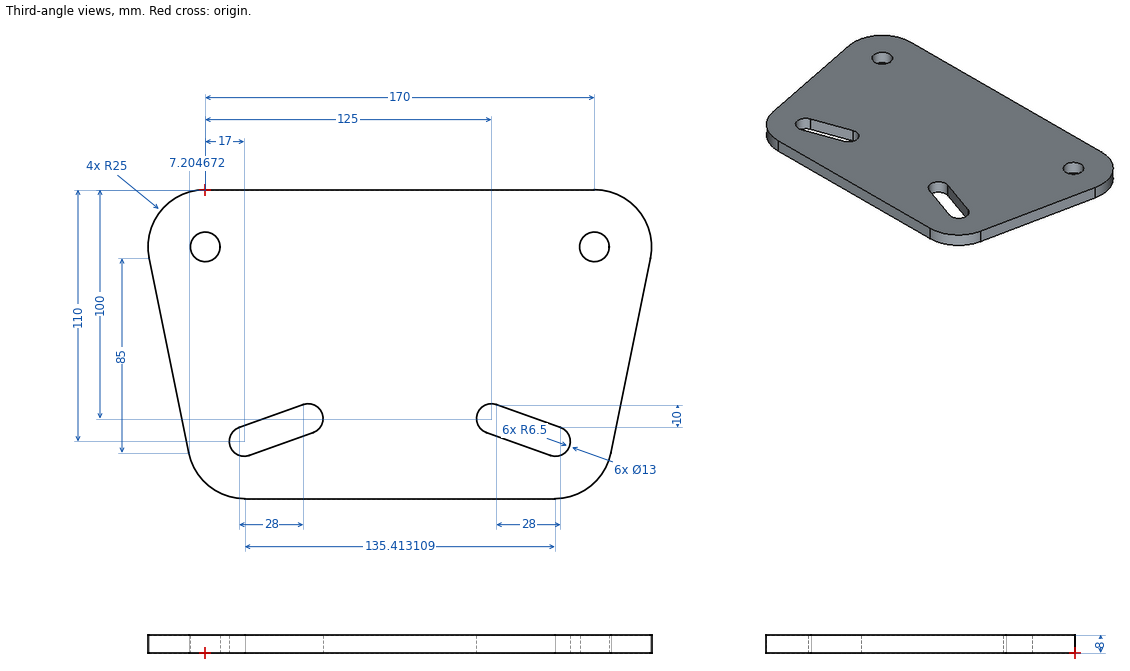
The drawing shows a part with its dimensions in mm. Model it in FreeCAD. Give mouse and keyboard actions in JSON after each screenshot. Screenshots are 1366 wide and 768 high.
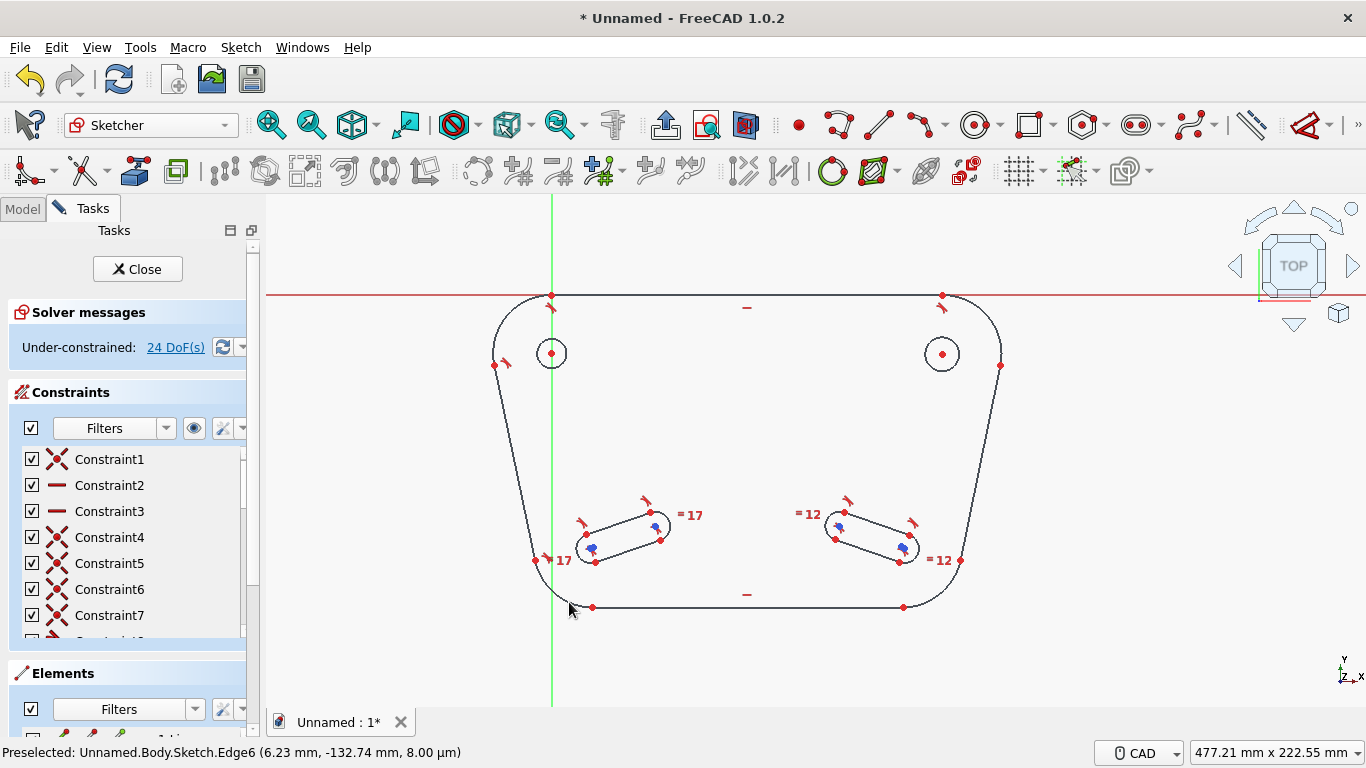
{"action": "left_click", "coordinate": [686, 608]}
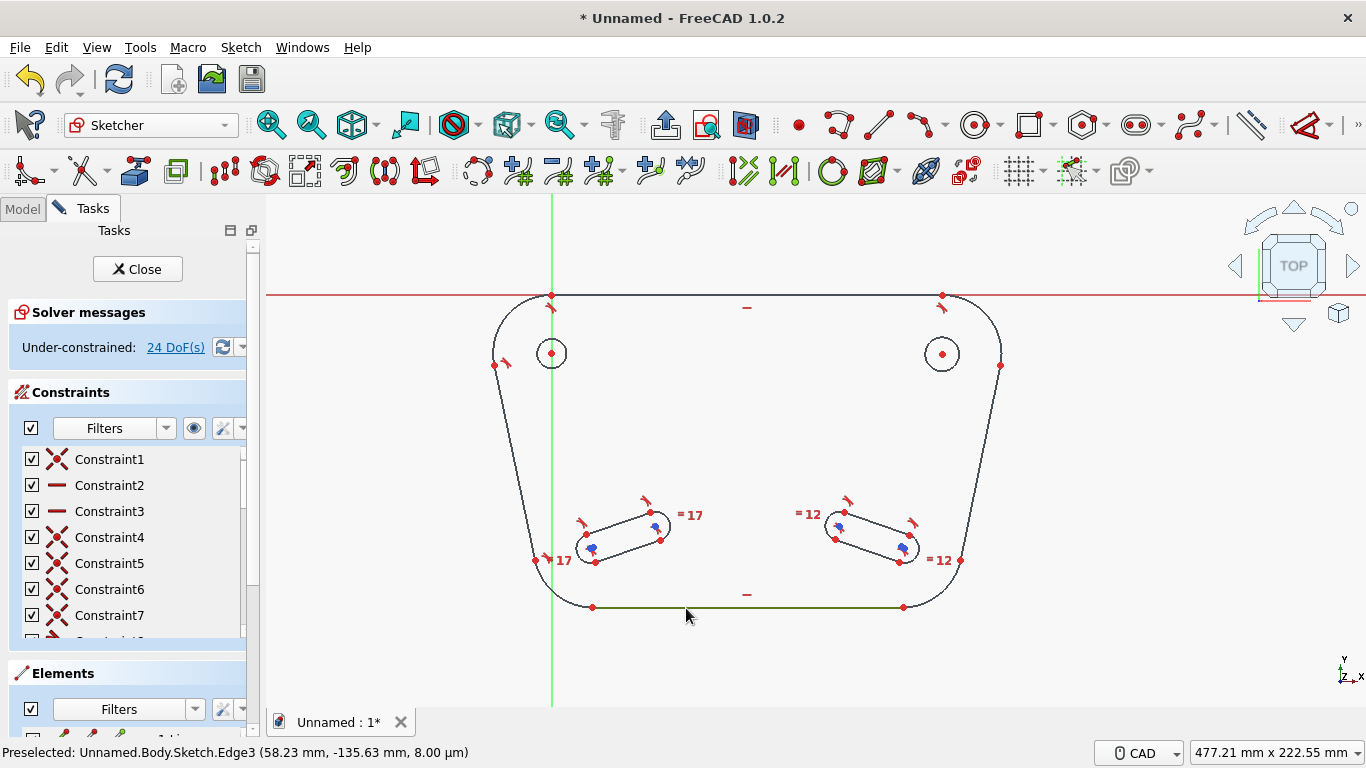
{"action": "left_click", "coordinate": [569, 602]}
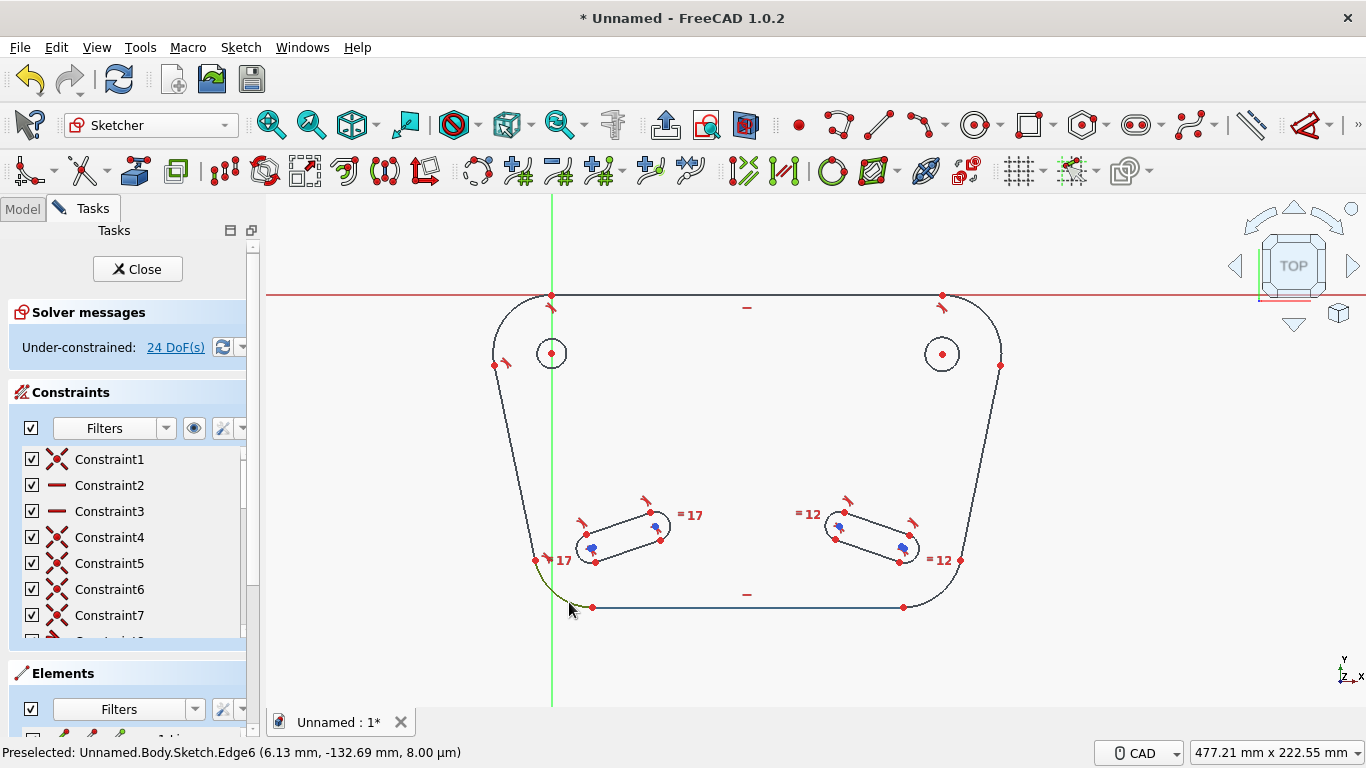
{"action": "key", "text": "t"}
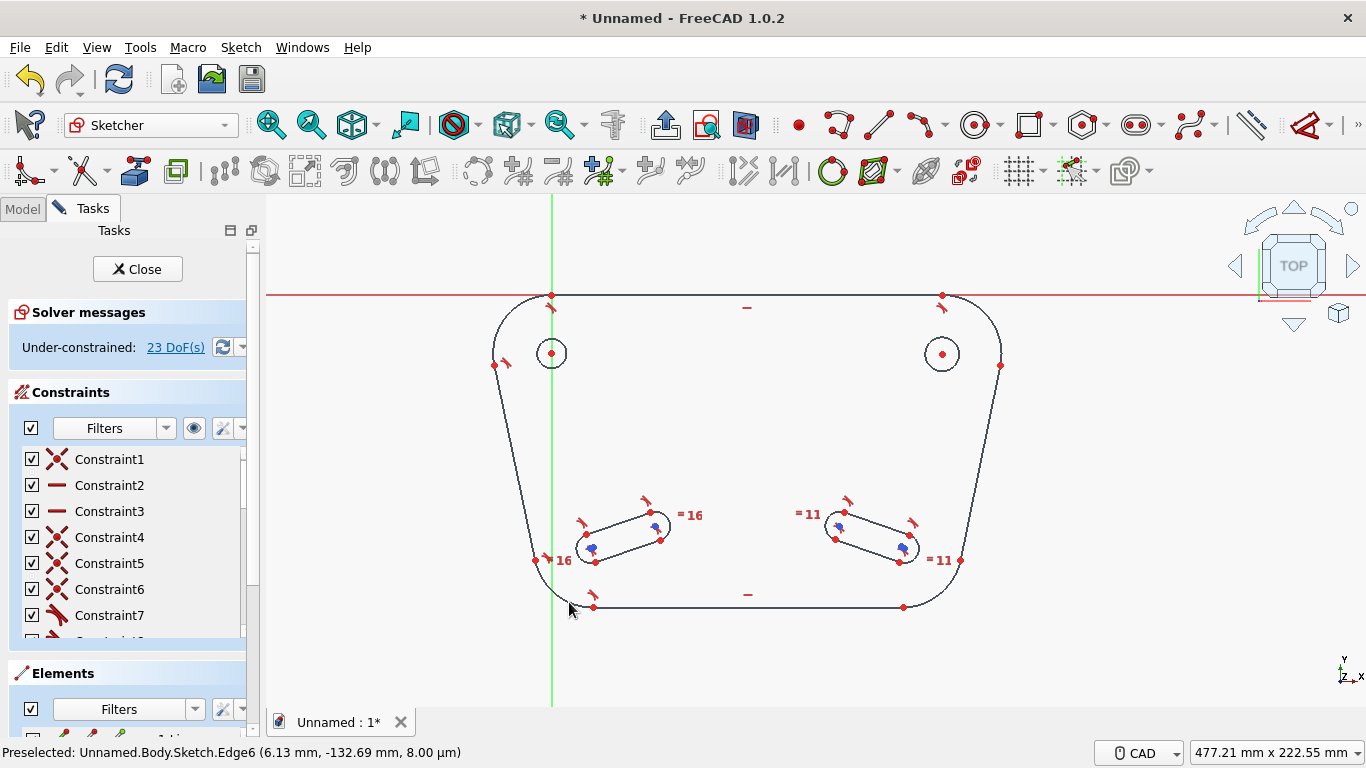
{"action": "left_click", "coordinate": [687, 608]}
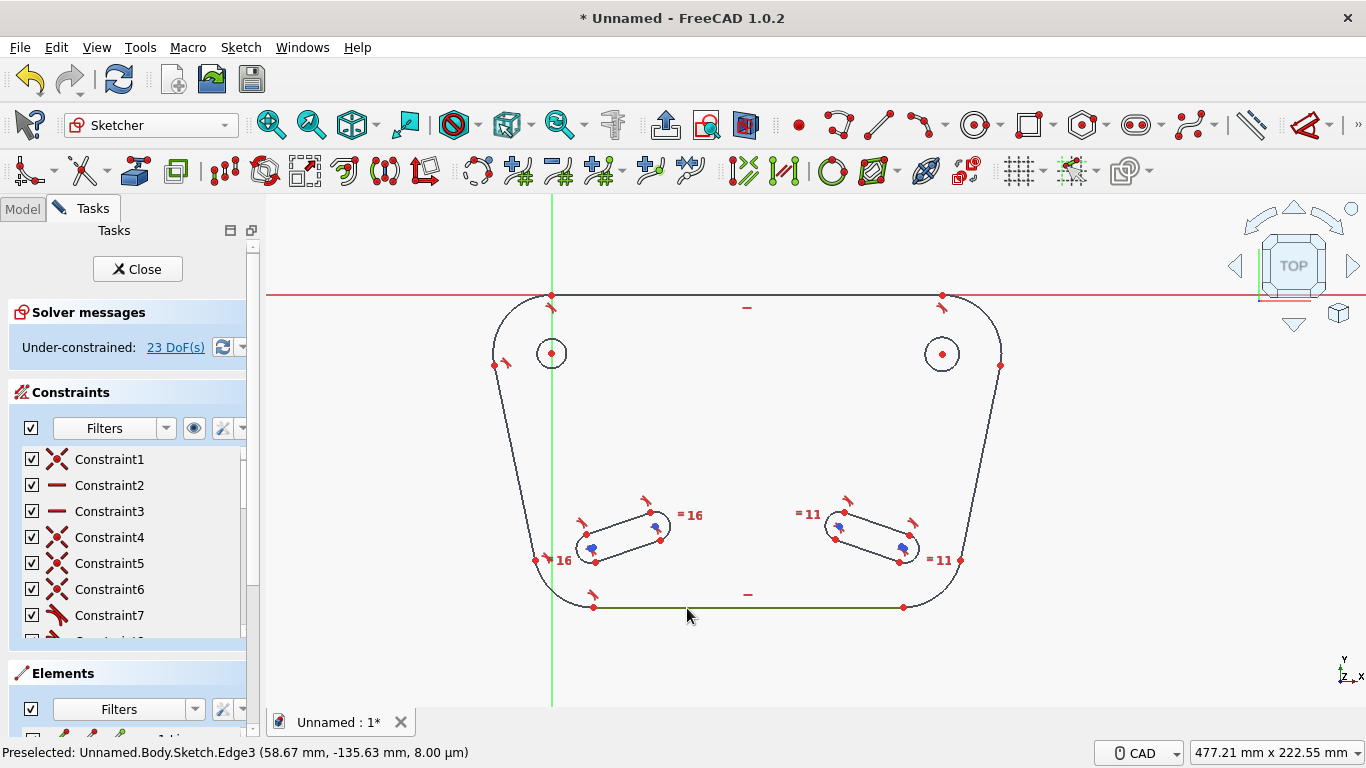
{"action": "left_click", "coordinate": [927, 602]}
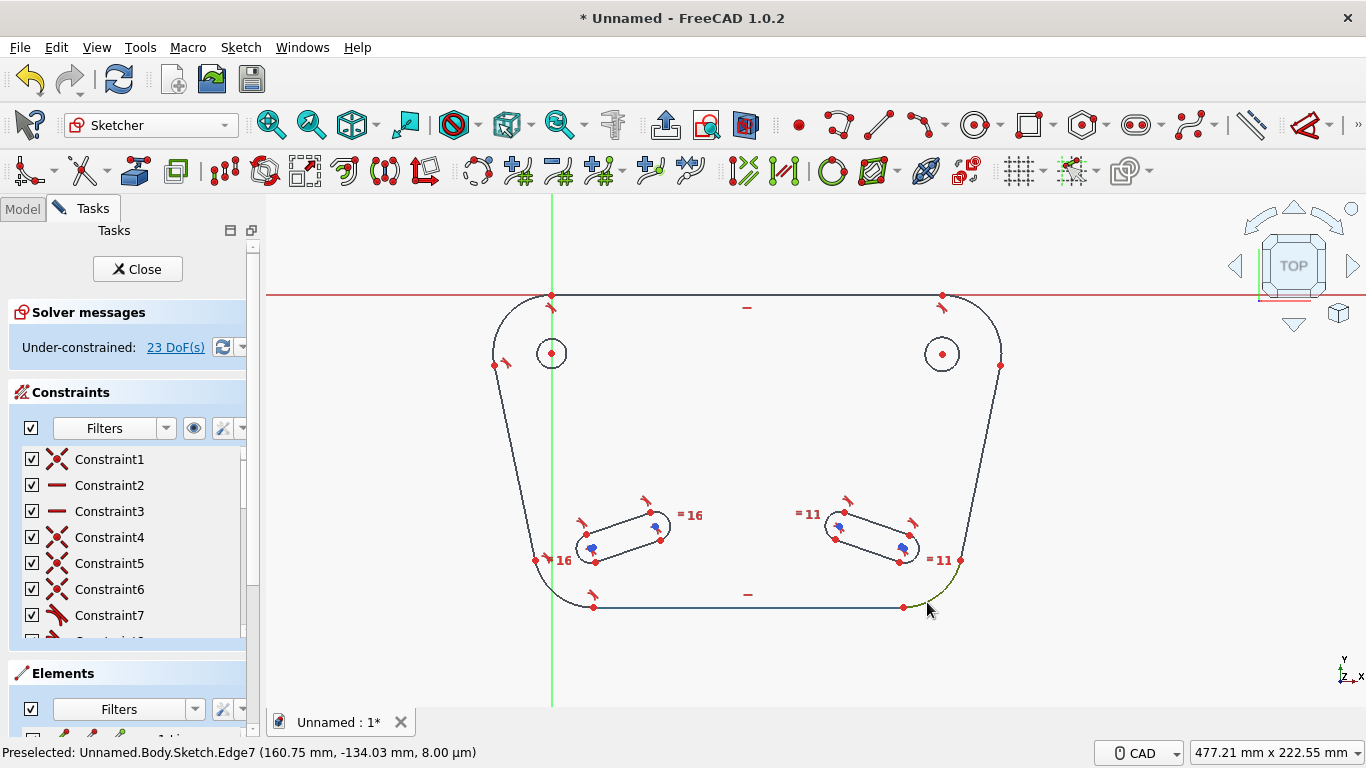
{"action": "key", "text": "t"}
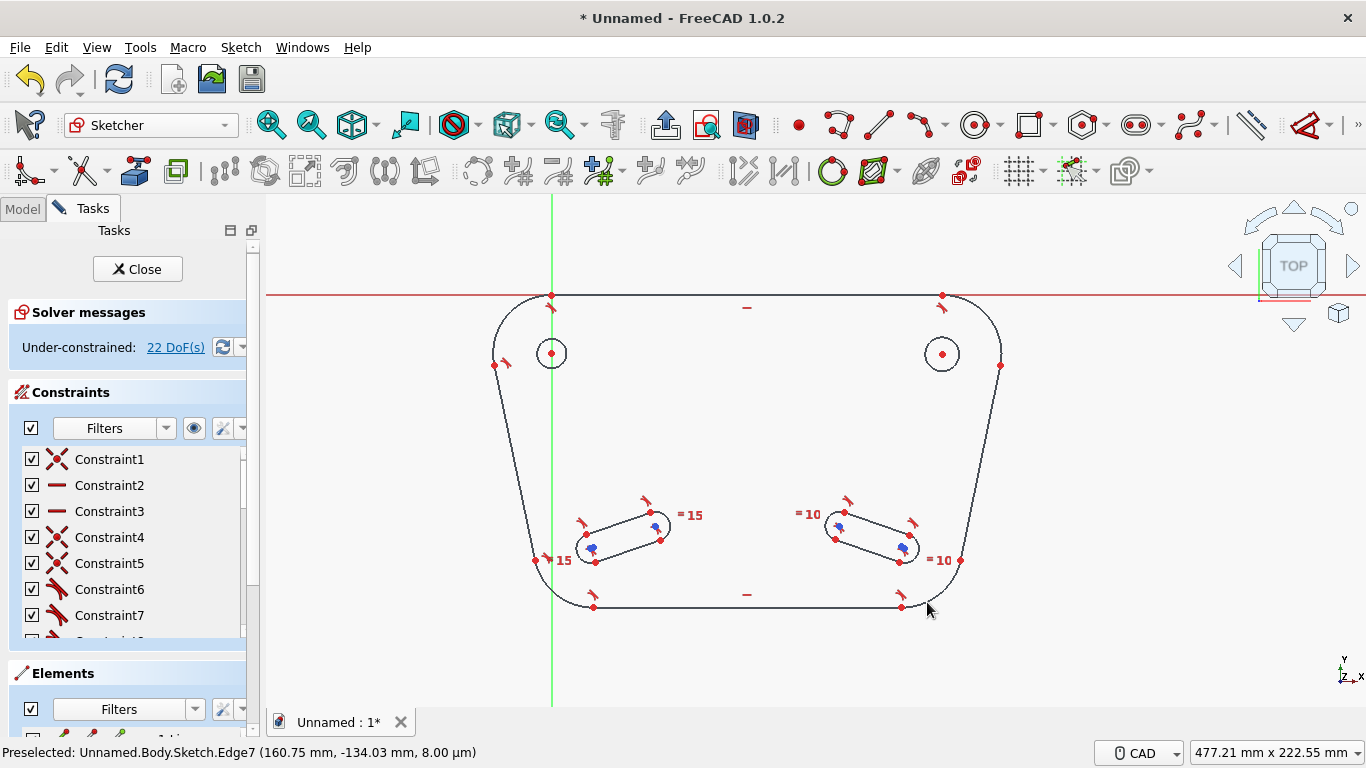
{"action": "left_click", "coordinate": [973, 502]}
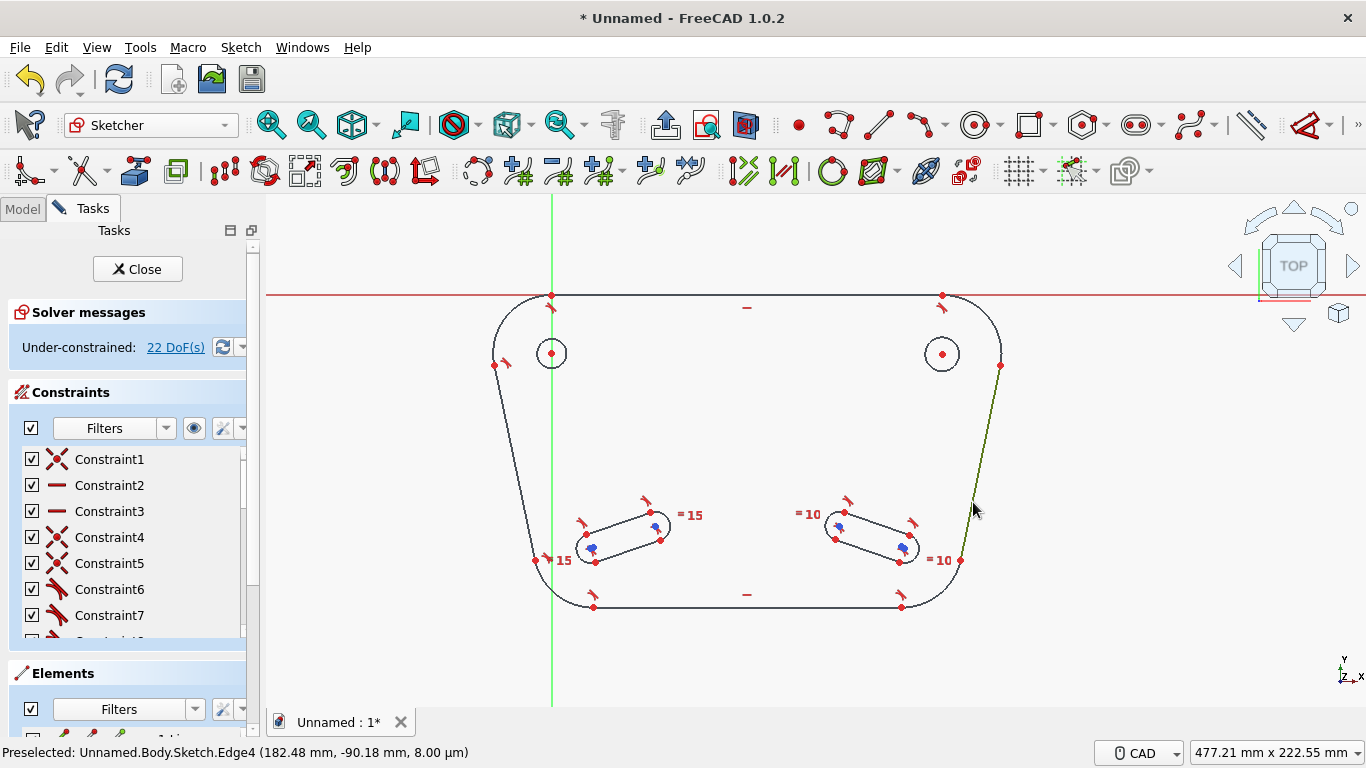
{"action": "left_click", "coordinate": [925, 603]}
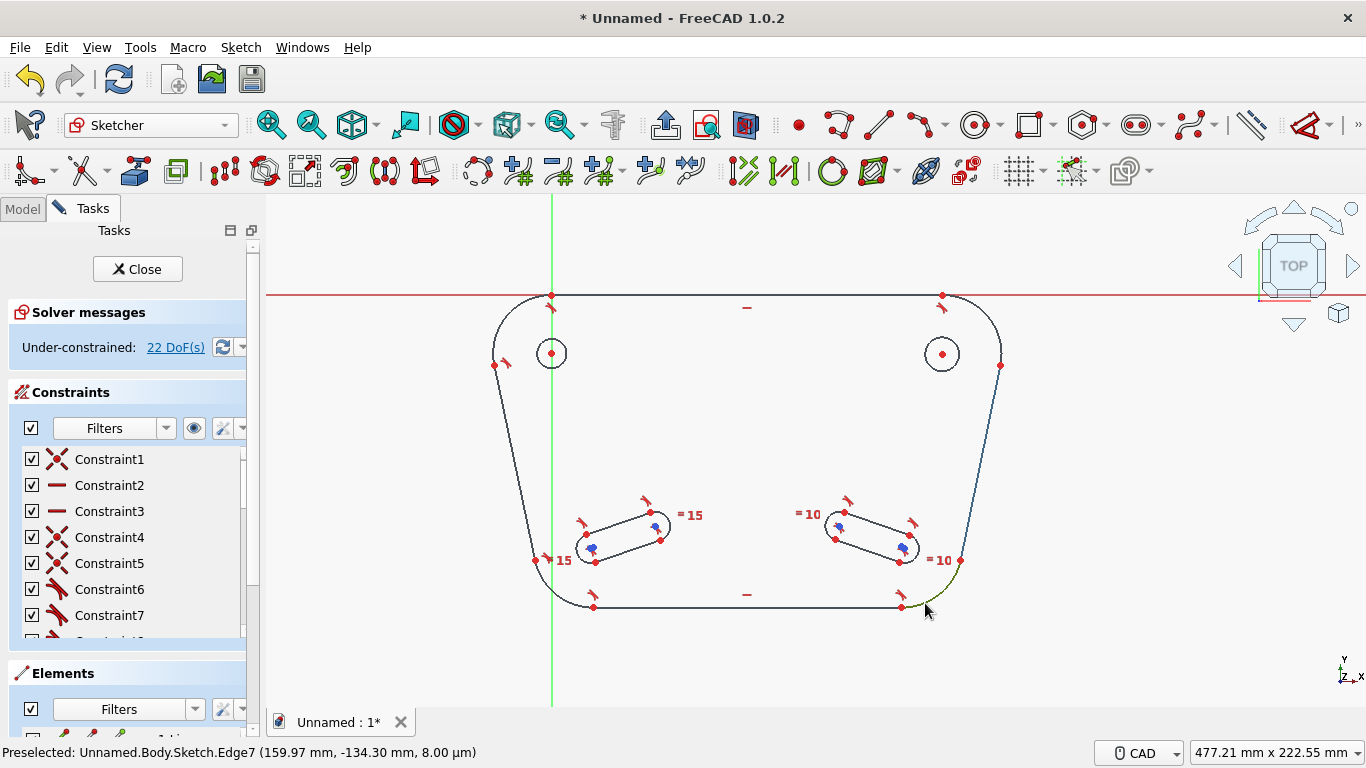
{"action": "key", "text": "t"}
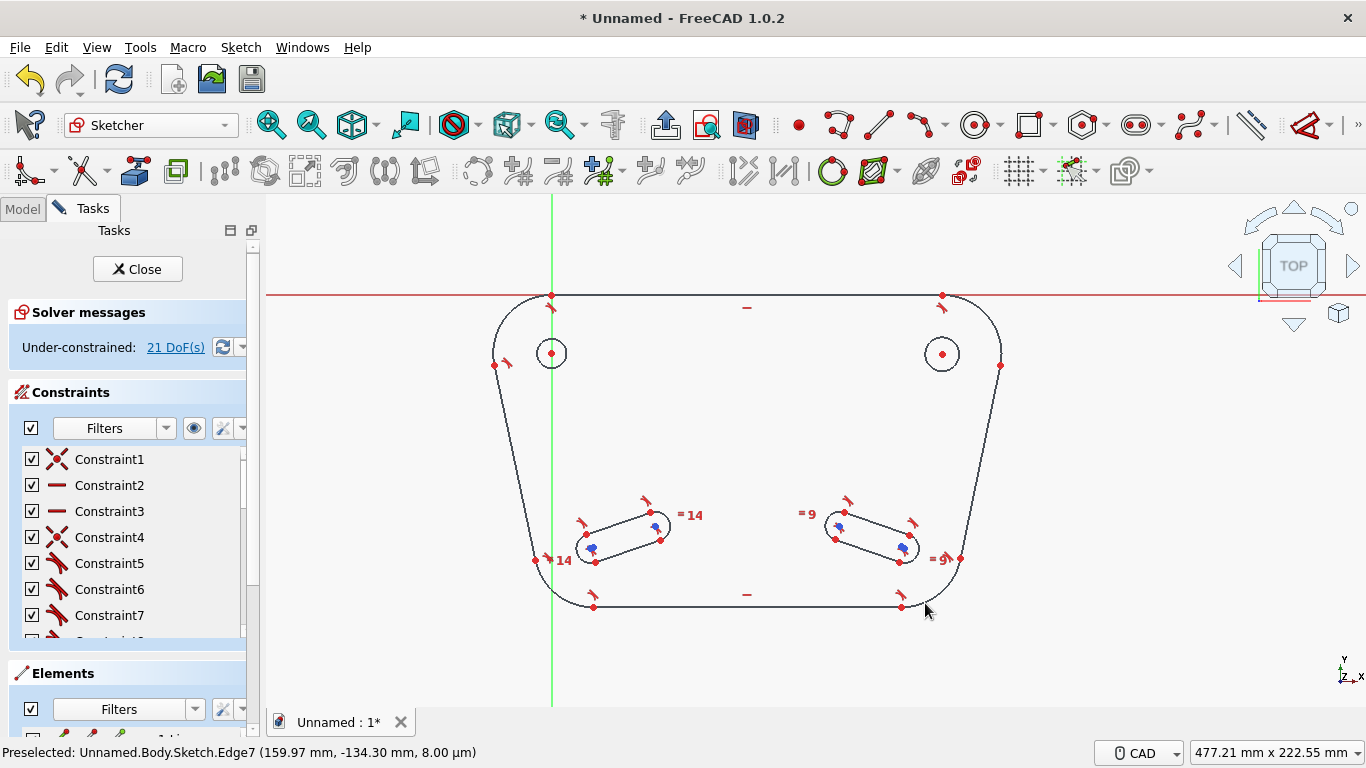
{"action": "left_click", "coordinate": [973, 501]}